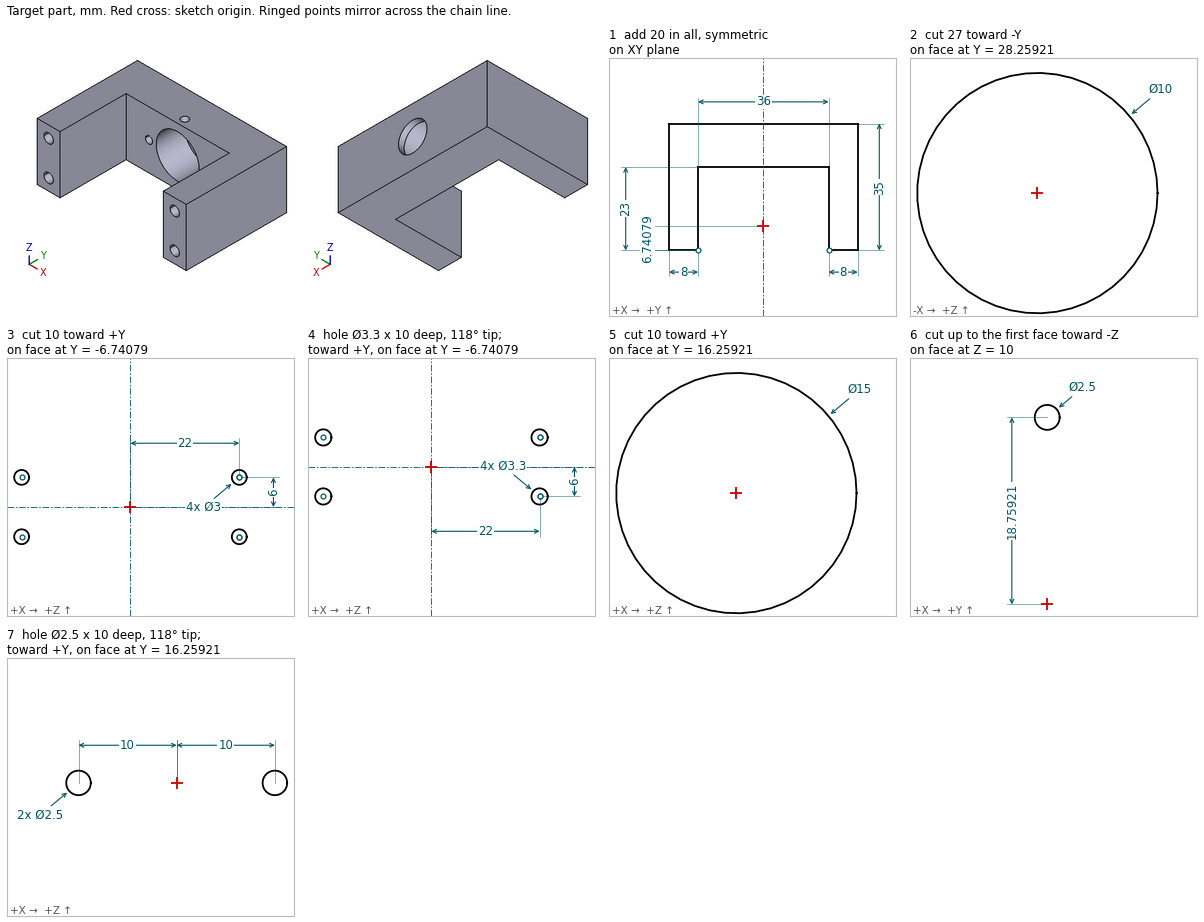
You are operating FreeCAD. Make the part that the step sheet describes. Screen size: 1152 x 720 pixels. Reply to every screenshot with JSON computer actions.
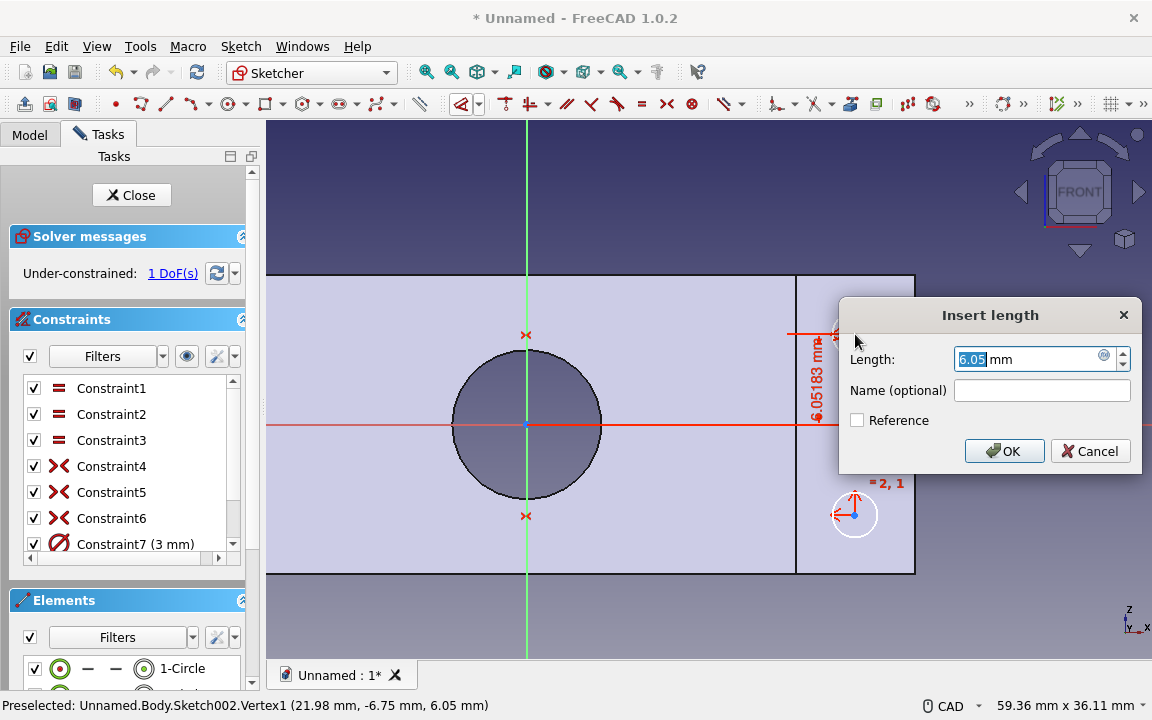
{"action": "type", "text": "6"}
{"action": "key", "text": "Return"}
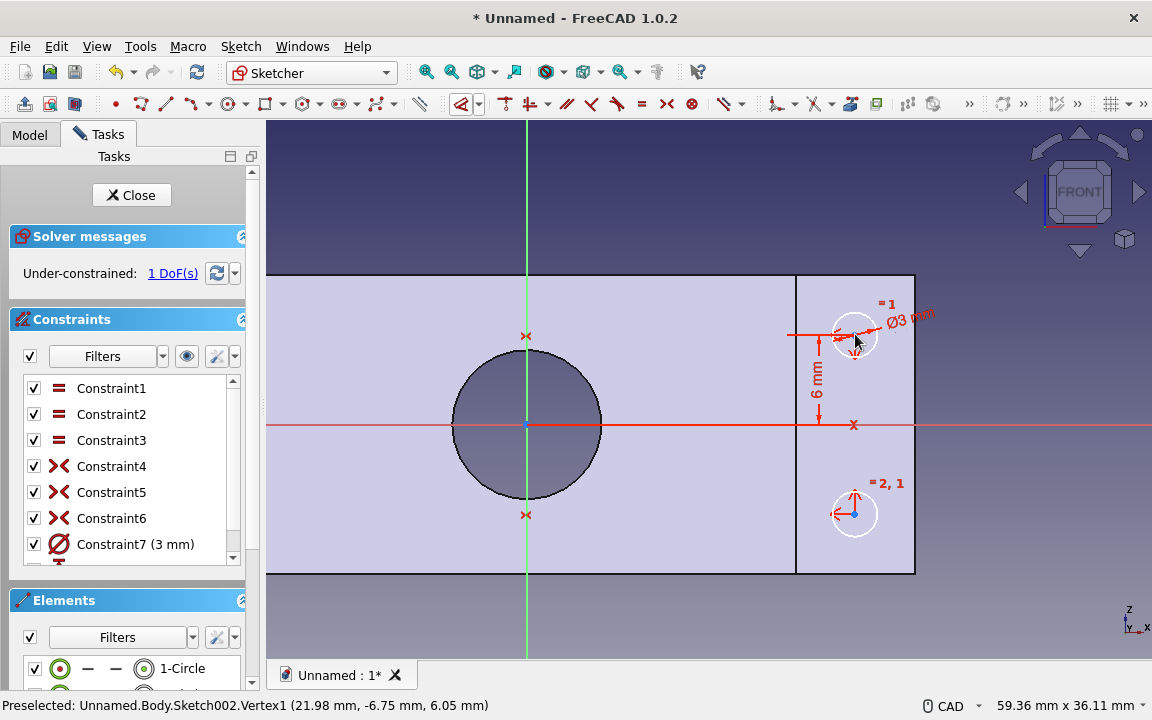
{"action": "left_click", "coordinate": [855, 335]}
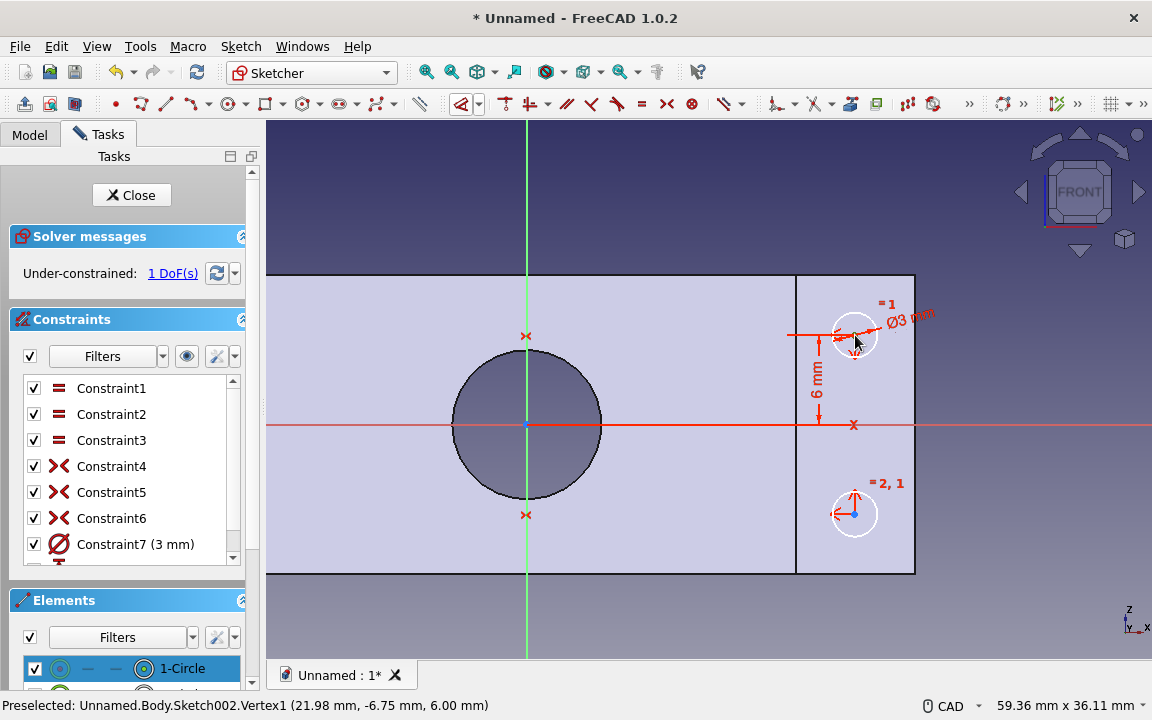
{"action": "left_click", "coordinate": [478, 104]}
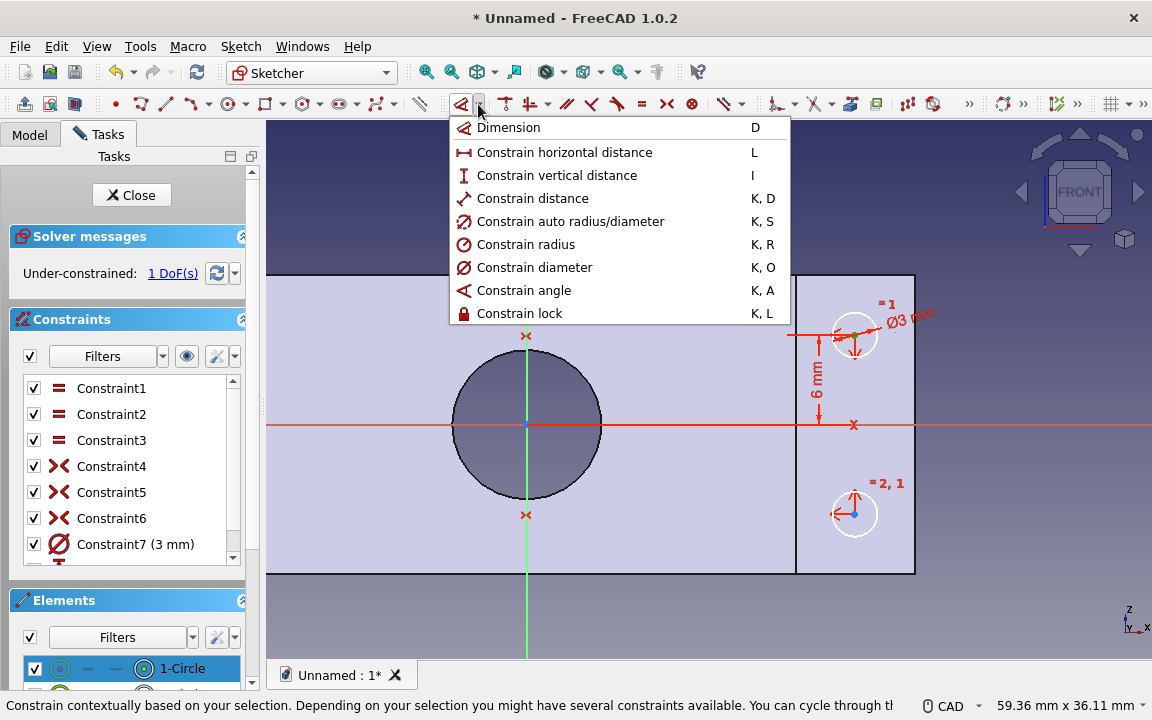
{"action": "left_click", "coordinate": [620, 152]}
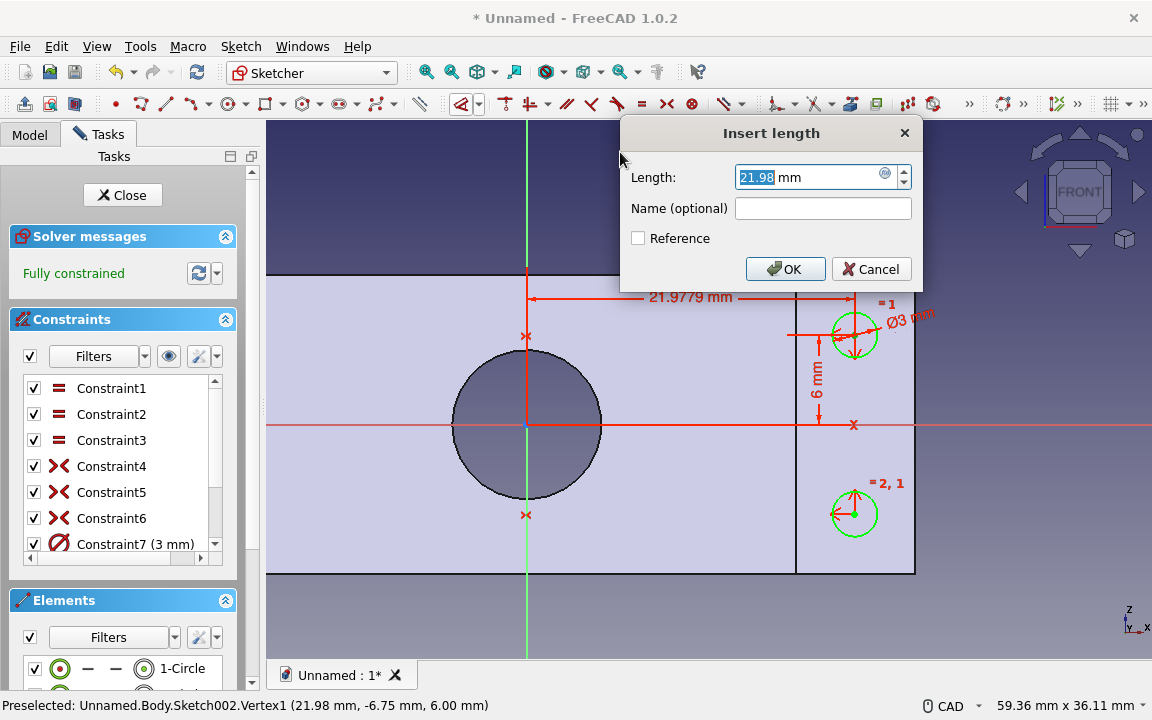
{"action": "type", "text": "22"}
{"action": "key", "text": "Return"}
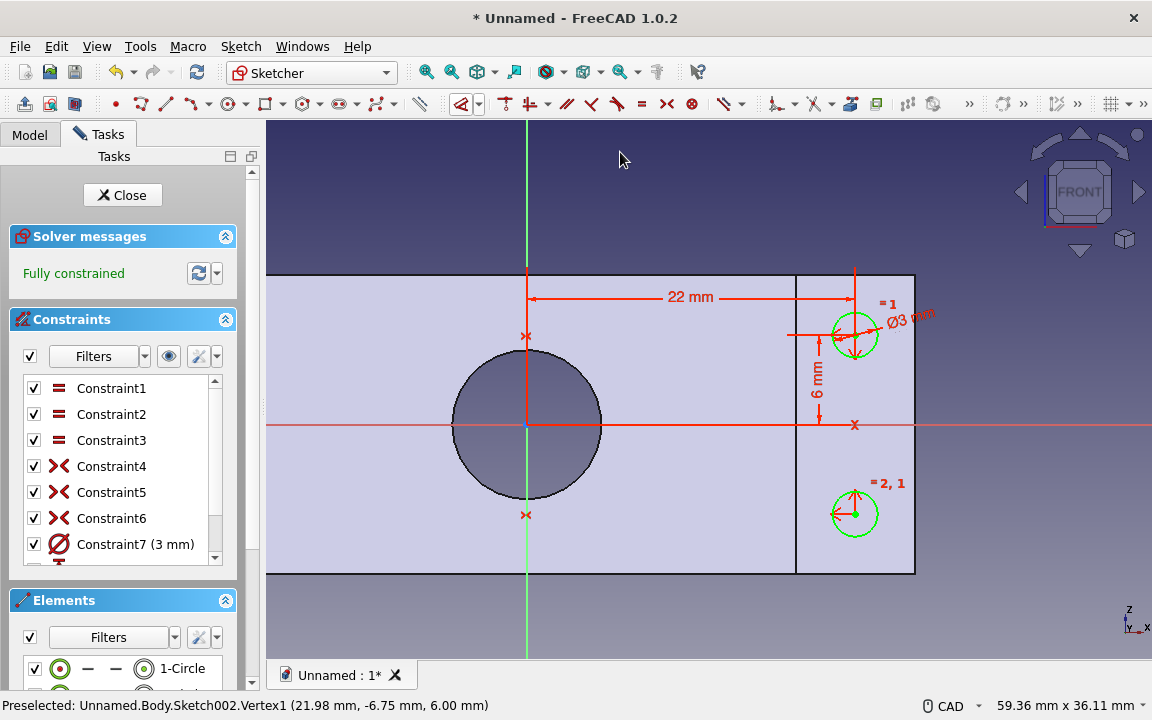
{"action": "left_click", "coordinate": [123, 195]}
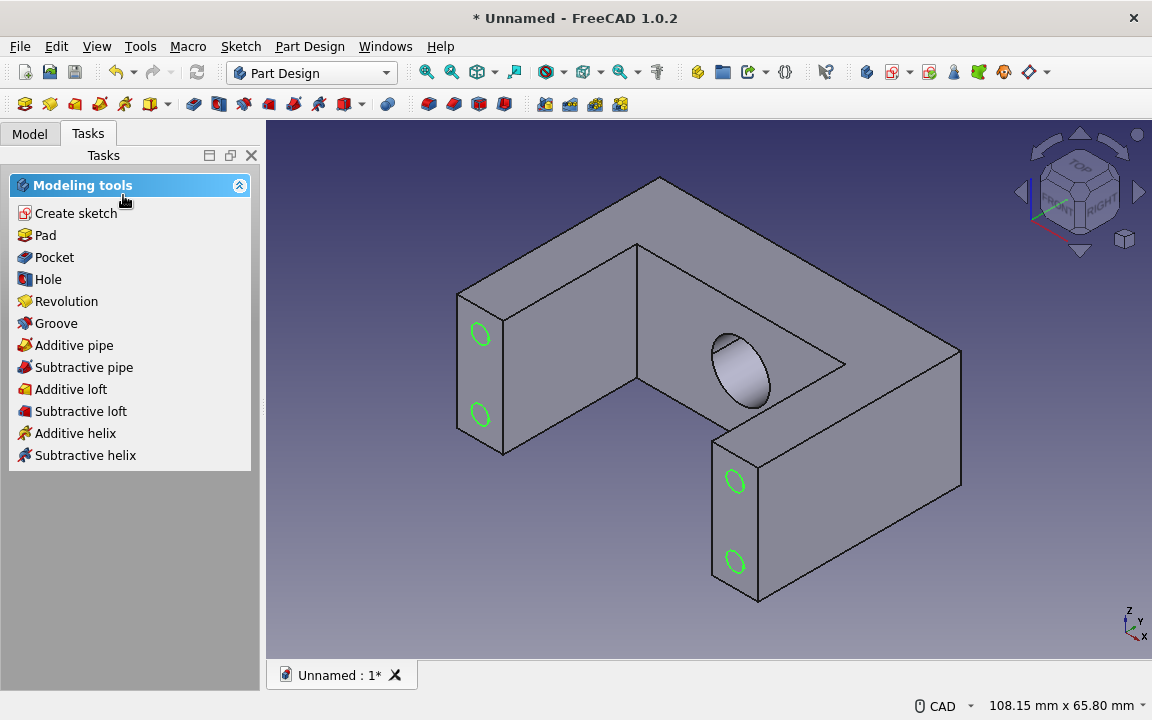
{"action": "left_click", "coordinate": [194, 104]}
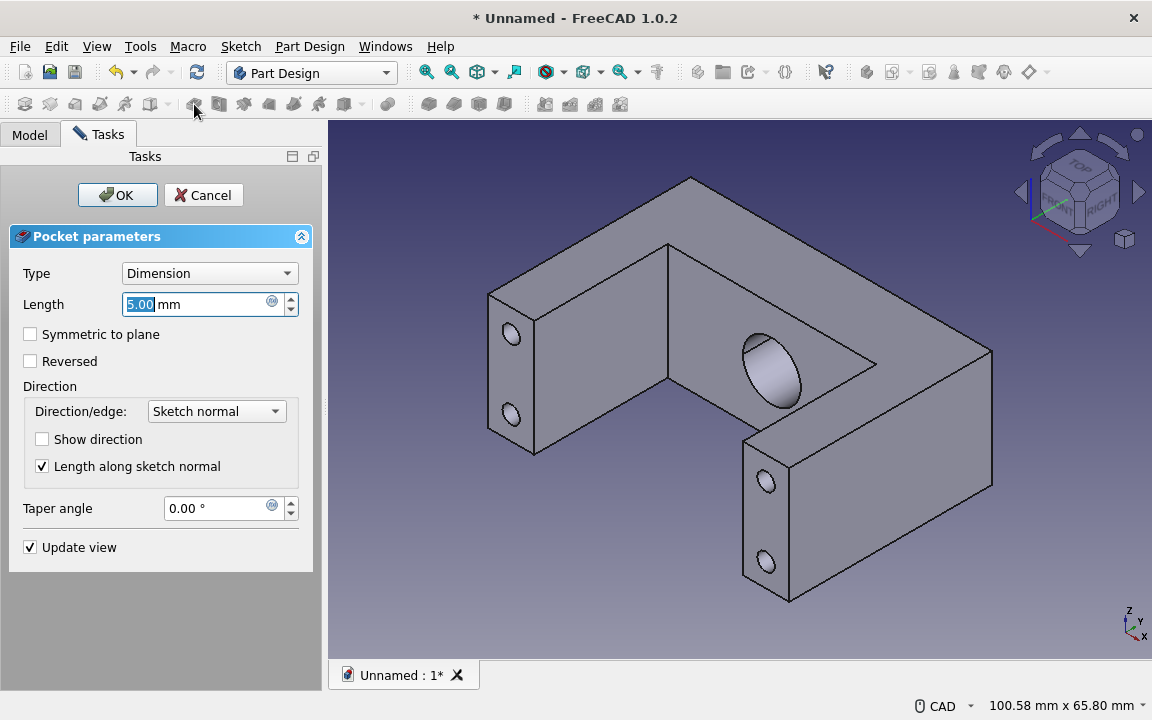
{"action": "type", "text": "10"}
{"action": "key", "text": "Tab"}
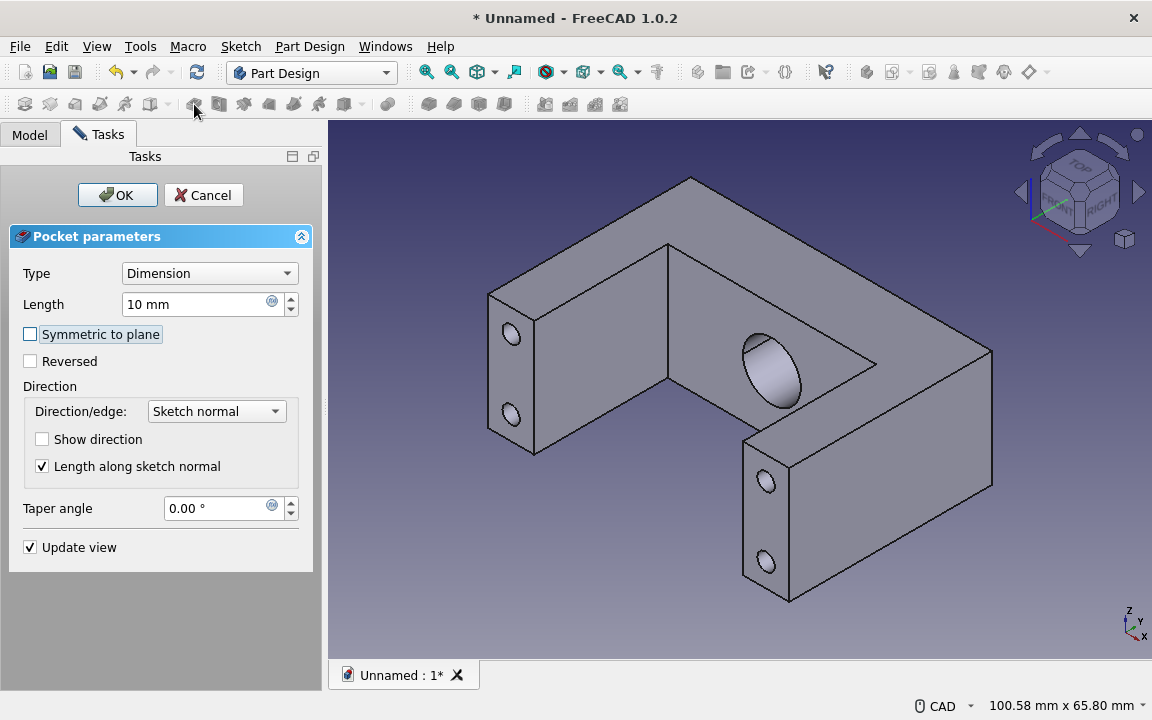
{"action": "left_click", "coordinate": [118, 195]}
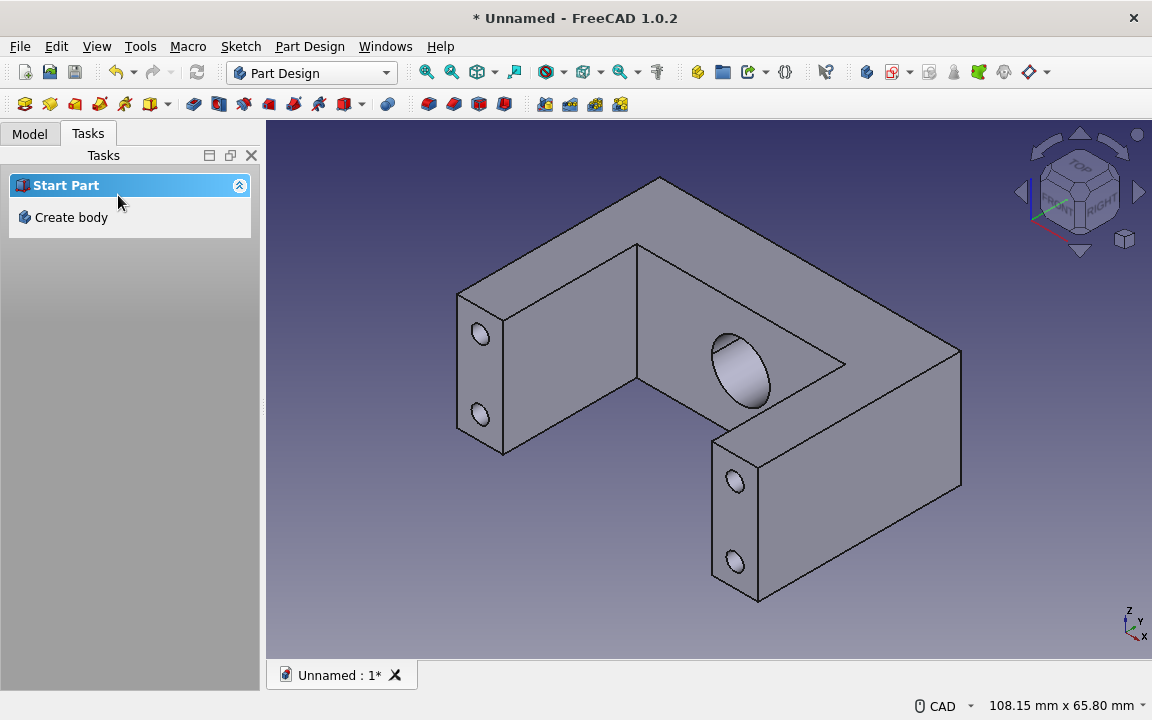
{"action": "left_click", "coordinate": [480, 373]}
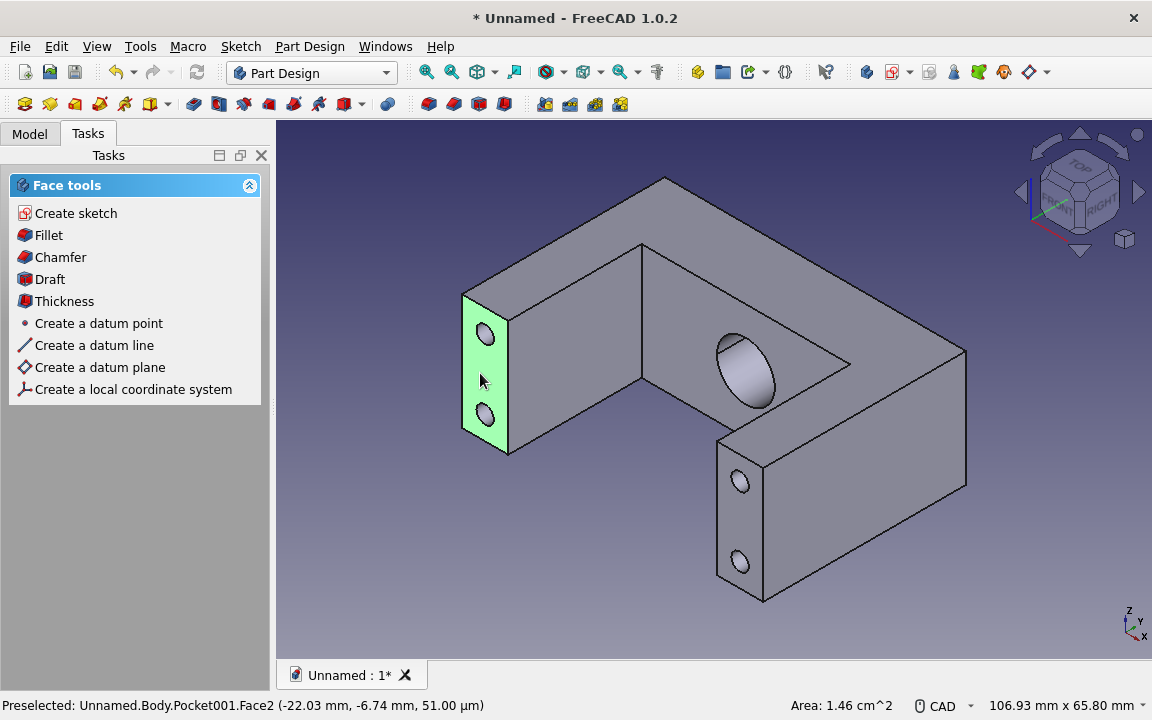
{"action": "left_click", "coordinate": [892, 72]}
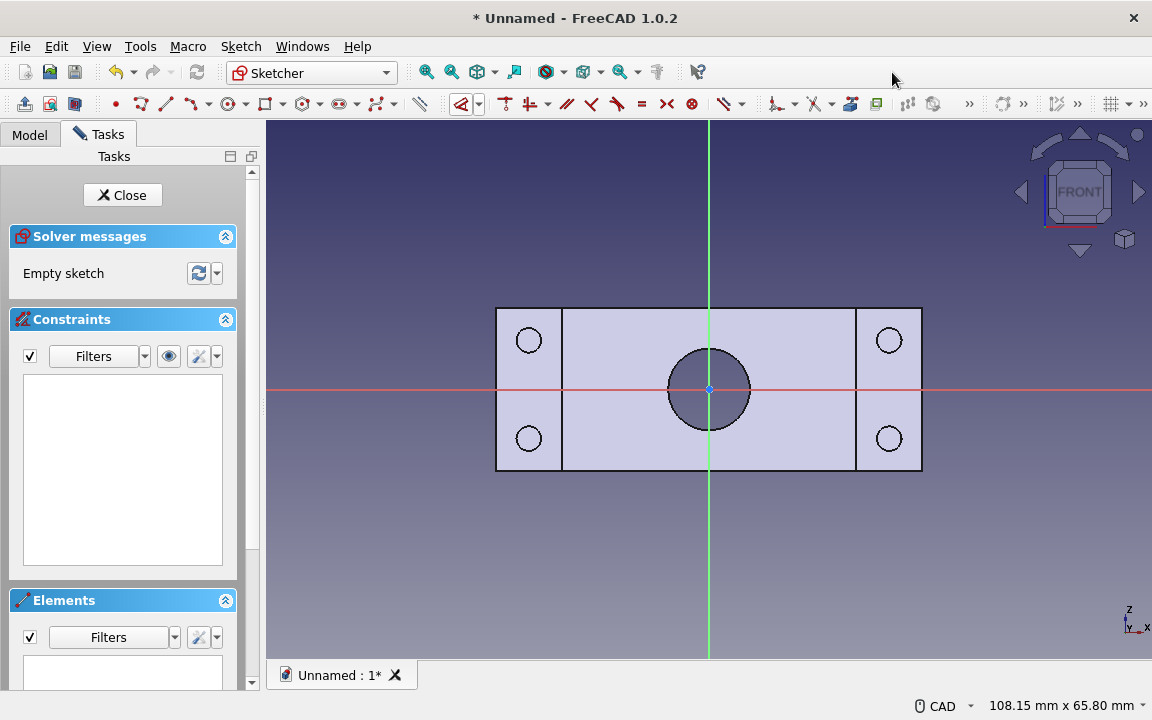
{"action": "key", "text": "g c"}